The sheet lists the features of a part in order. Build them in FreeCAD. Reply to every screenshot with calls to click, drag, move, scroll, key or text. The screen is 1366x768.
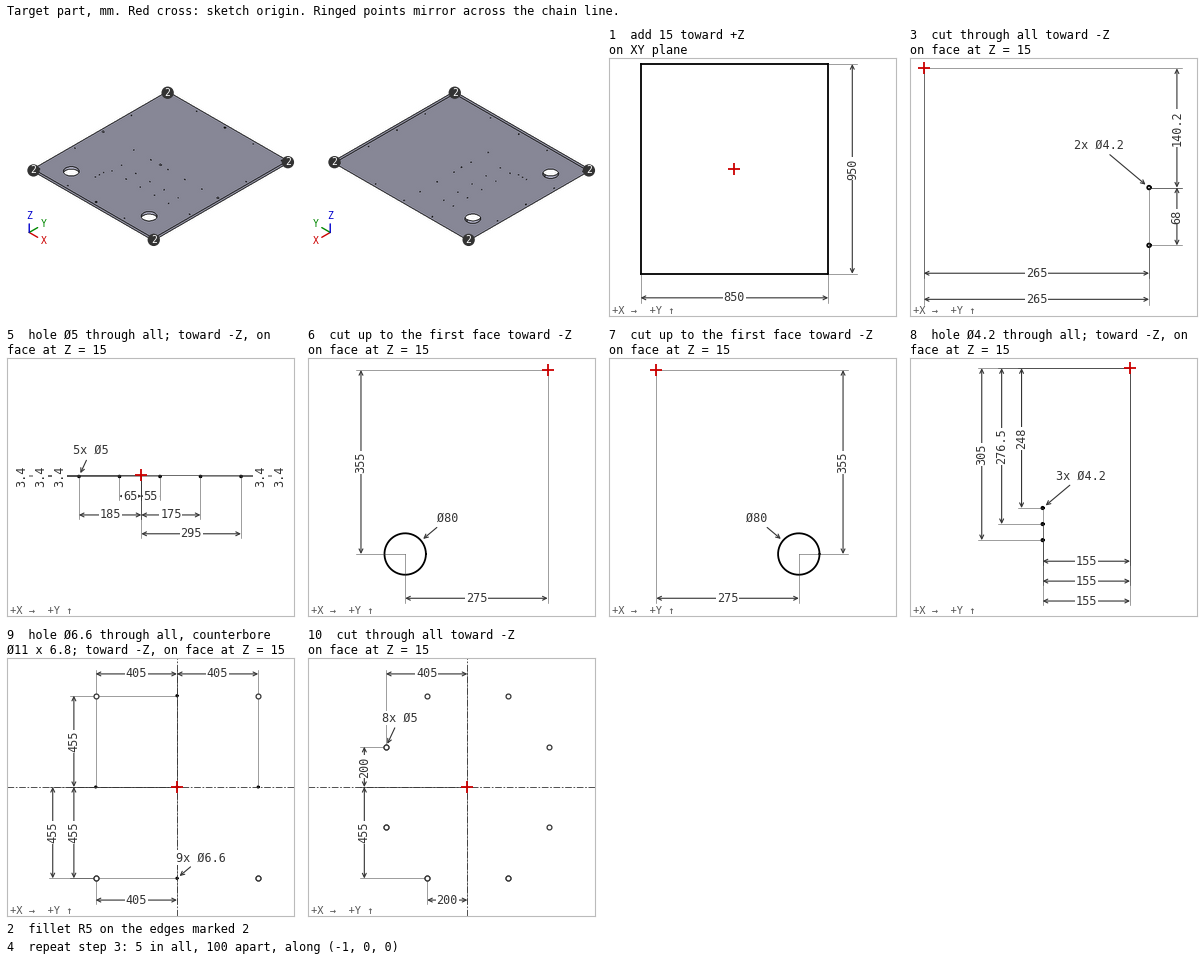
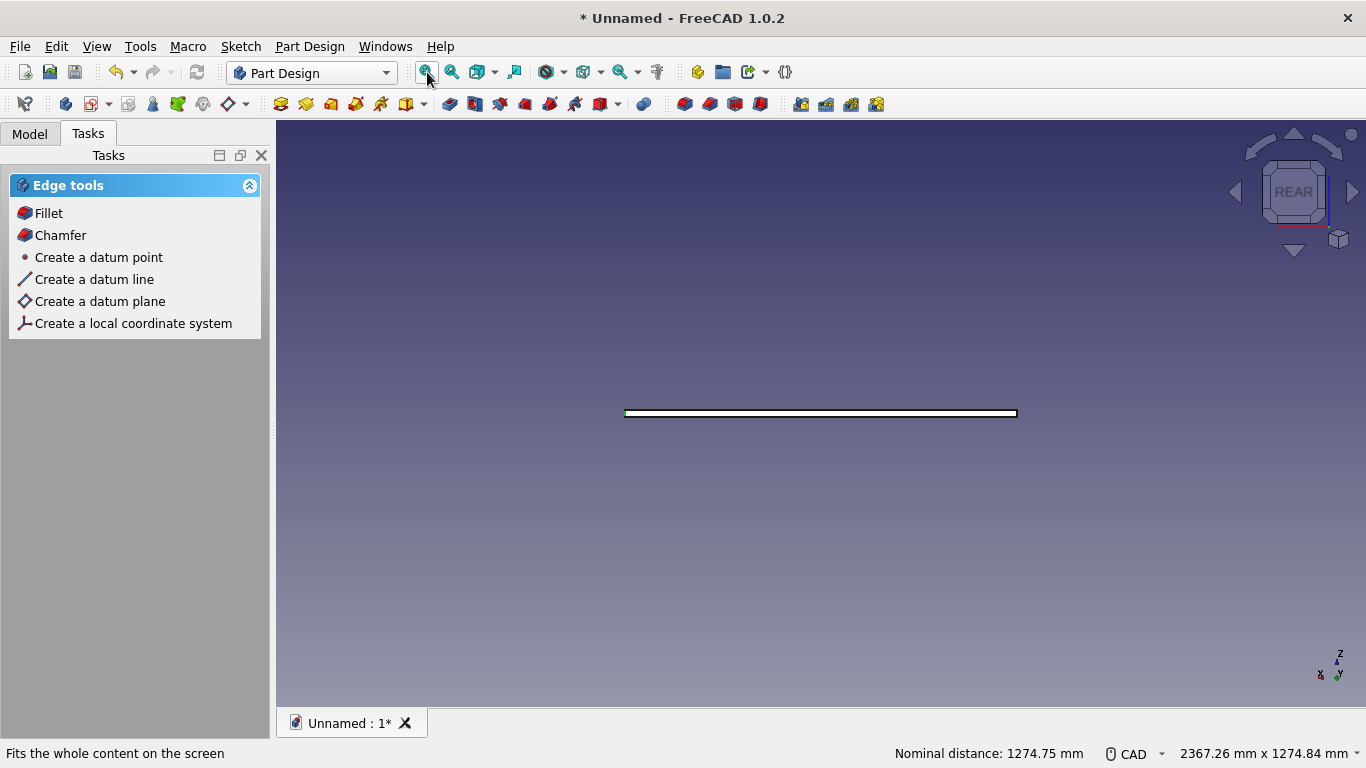
click(427, 72)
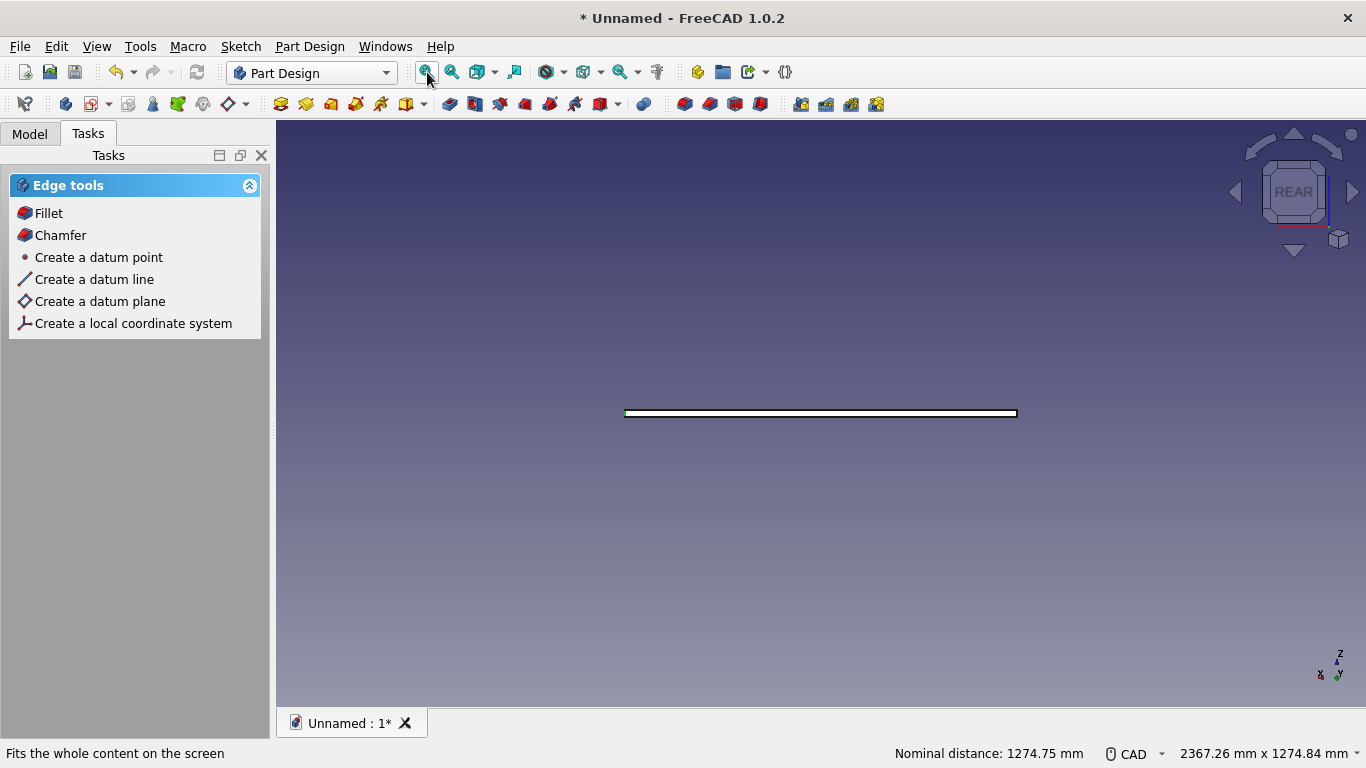
scroll(1017, 413, up, 9)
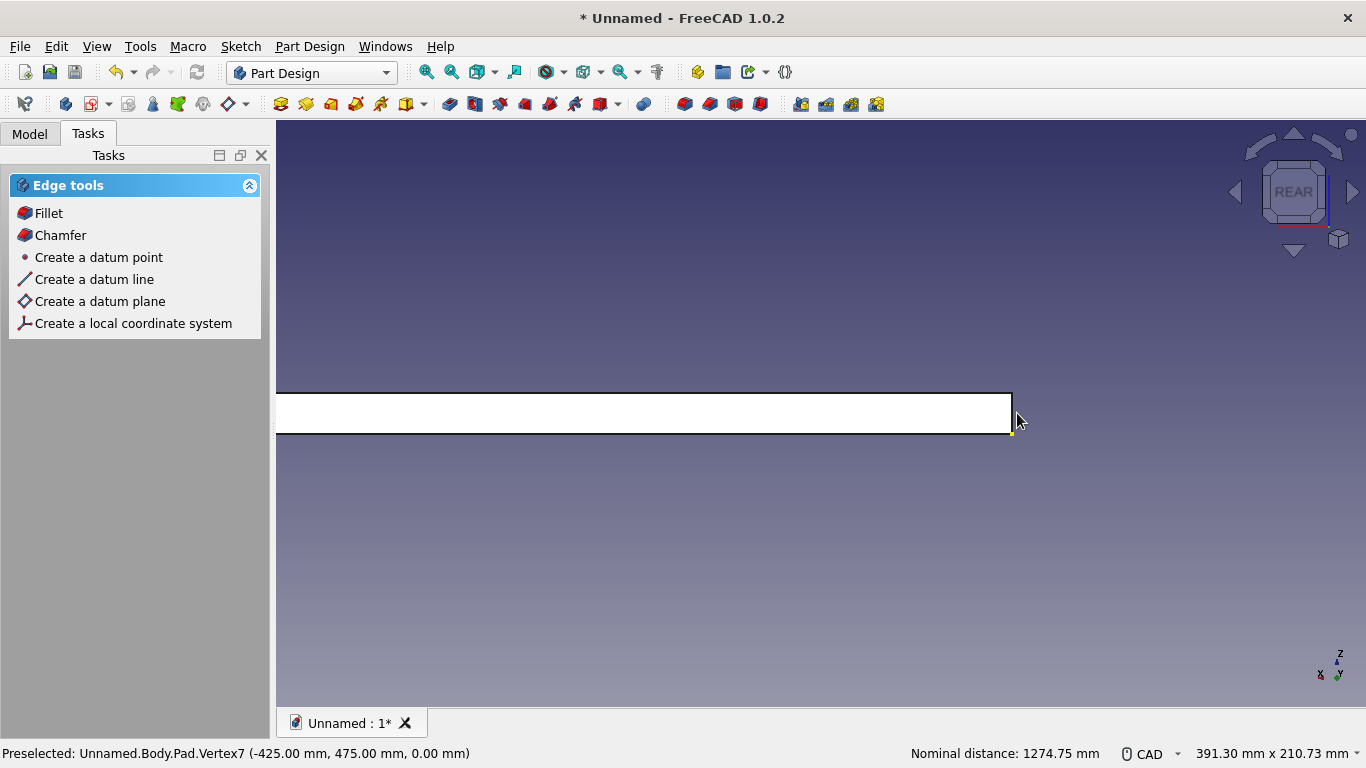
click(1012, 413, ctrl)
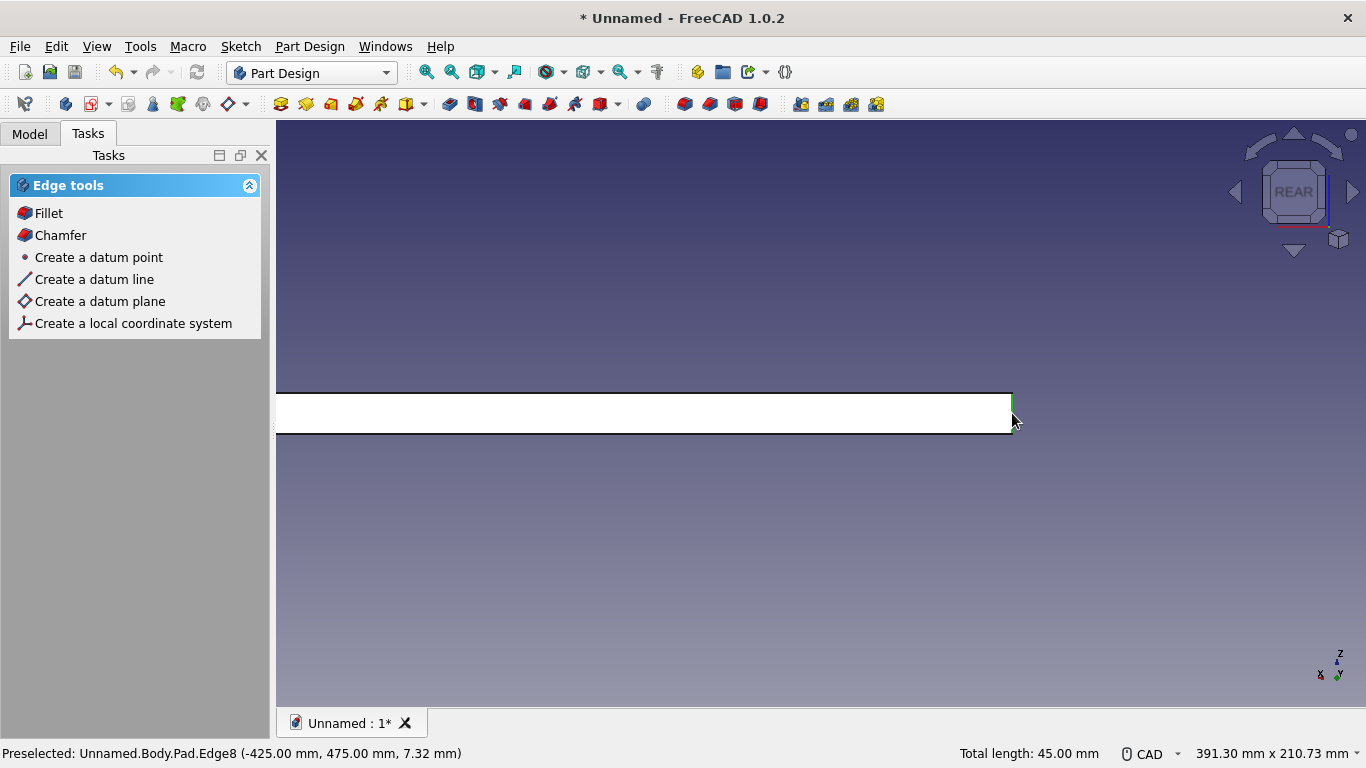
click(427, 72)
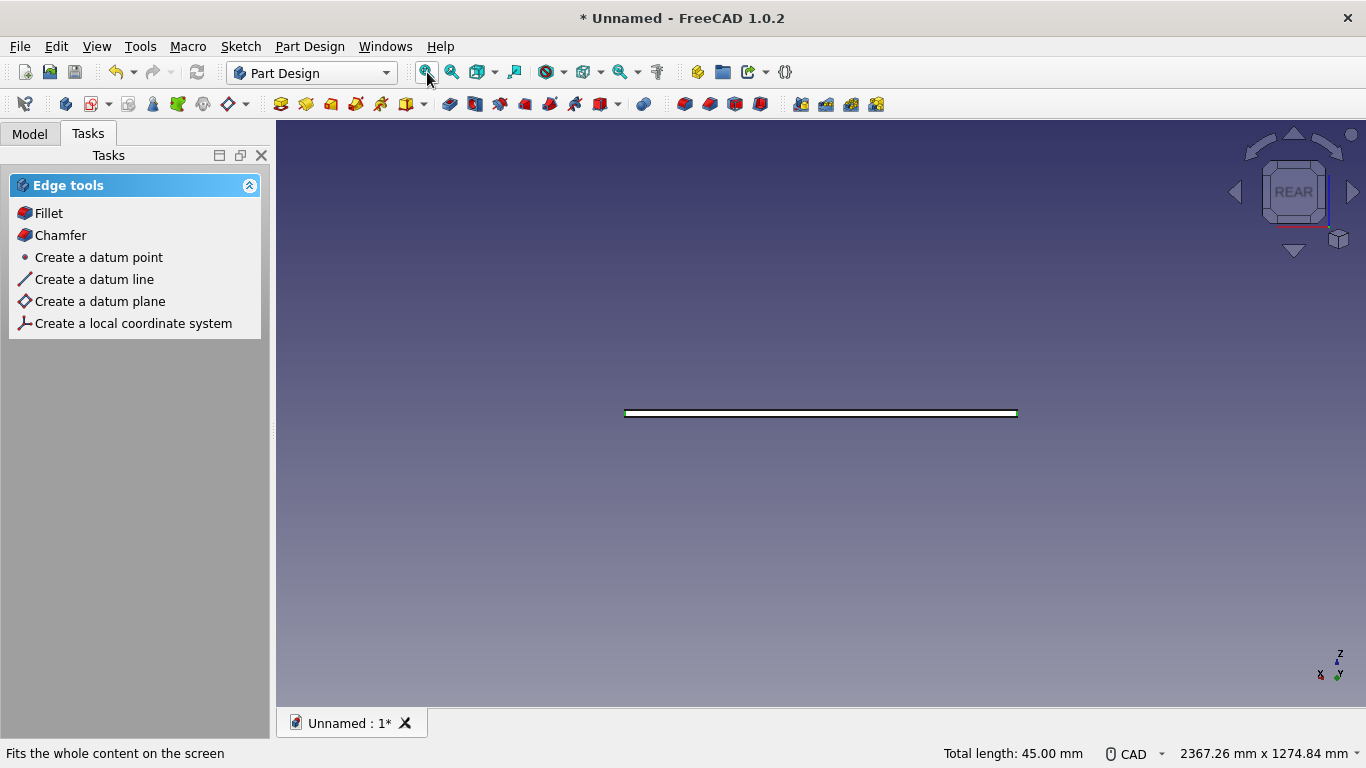
key(6)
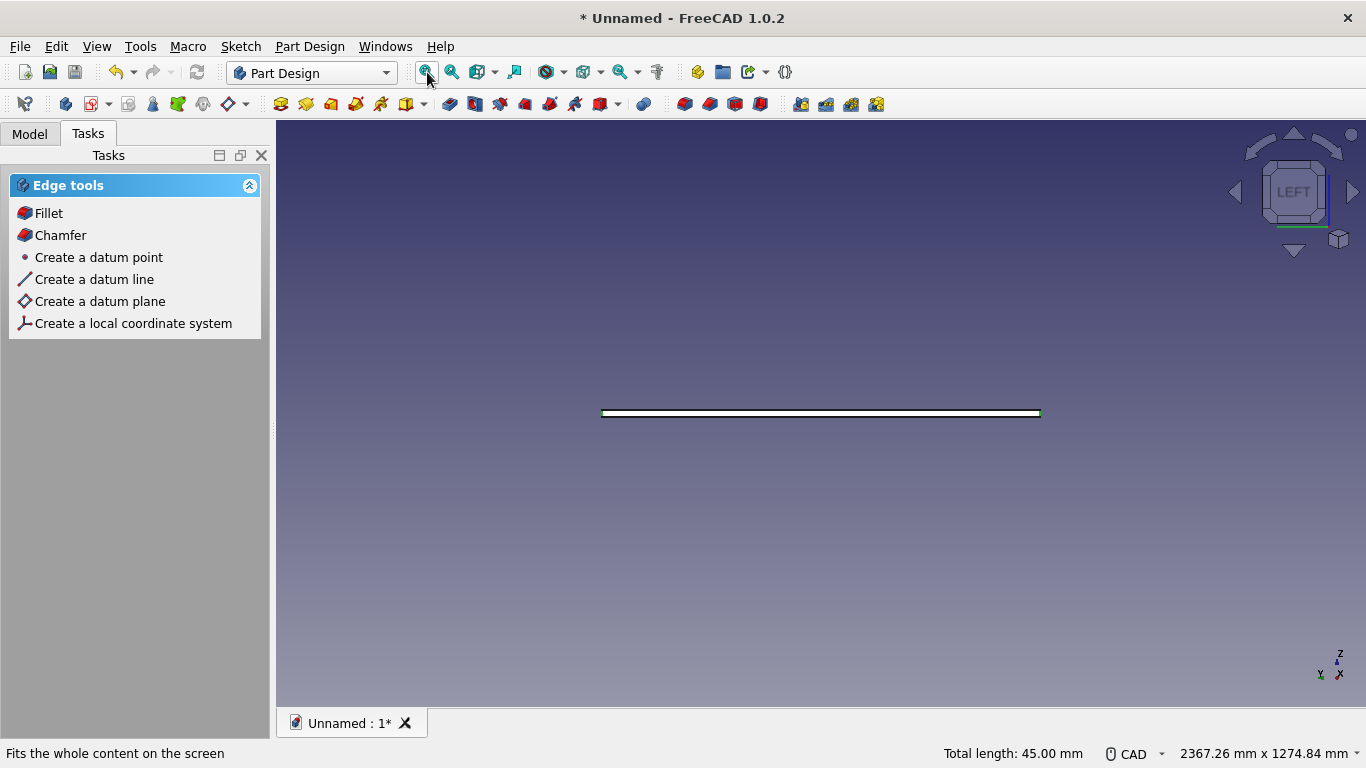
click(427, 72)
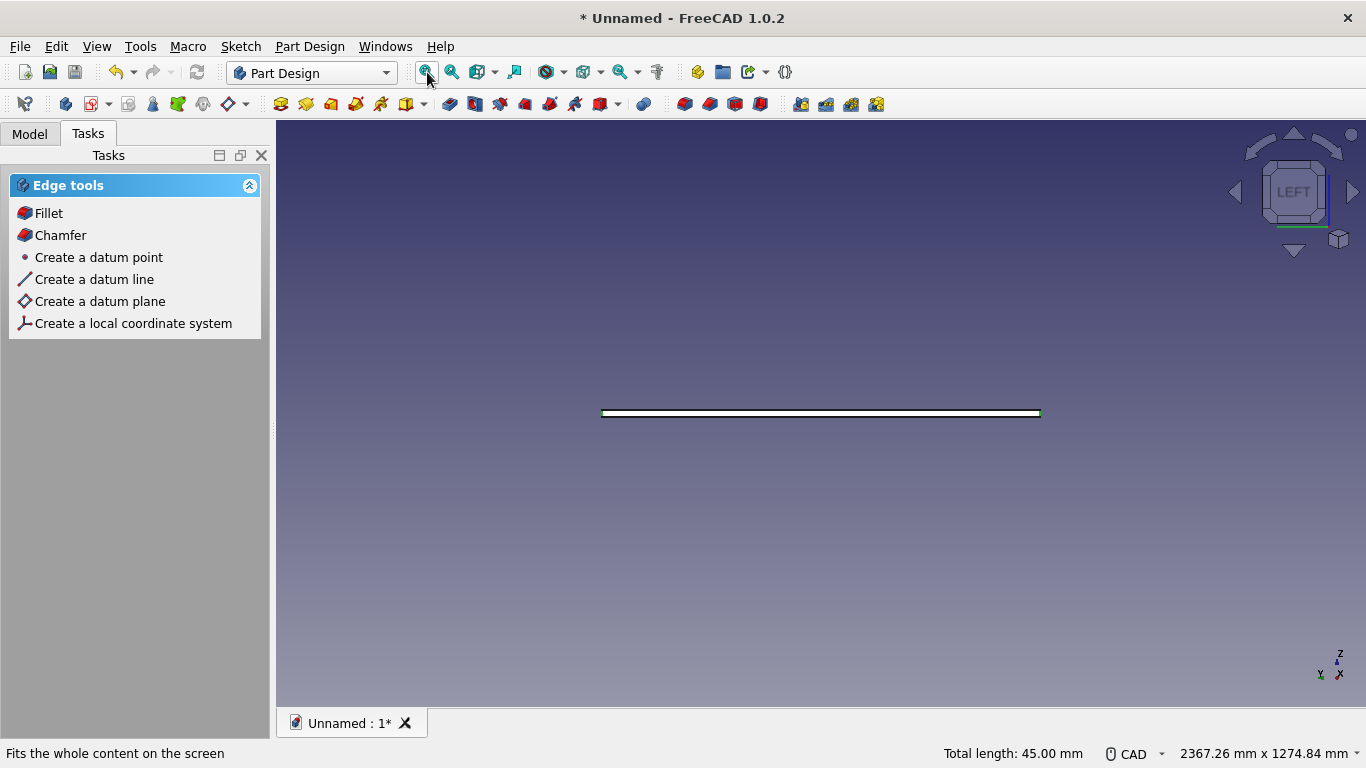
scroll(1040, 412, up, 9)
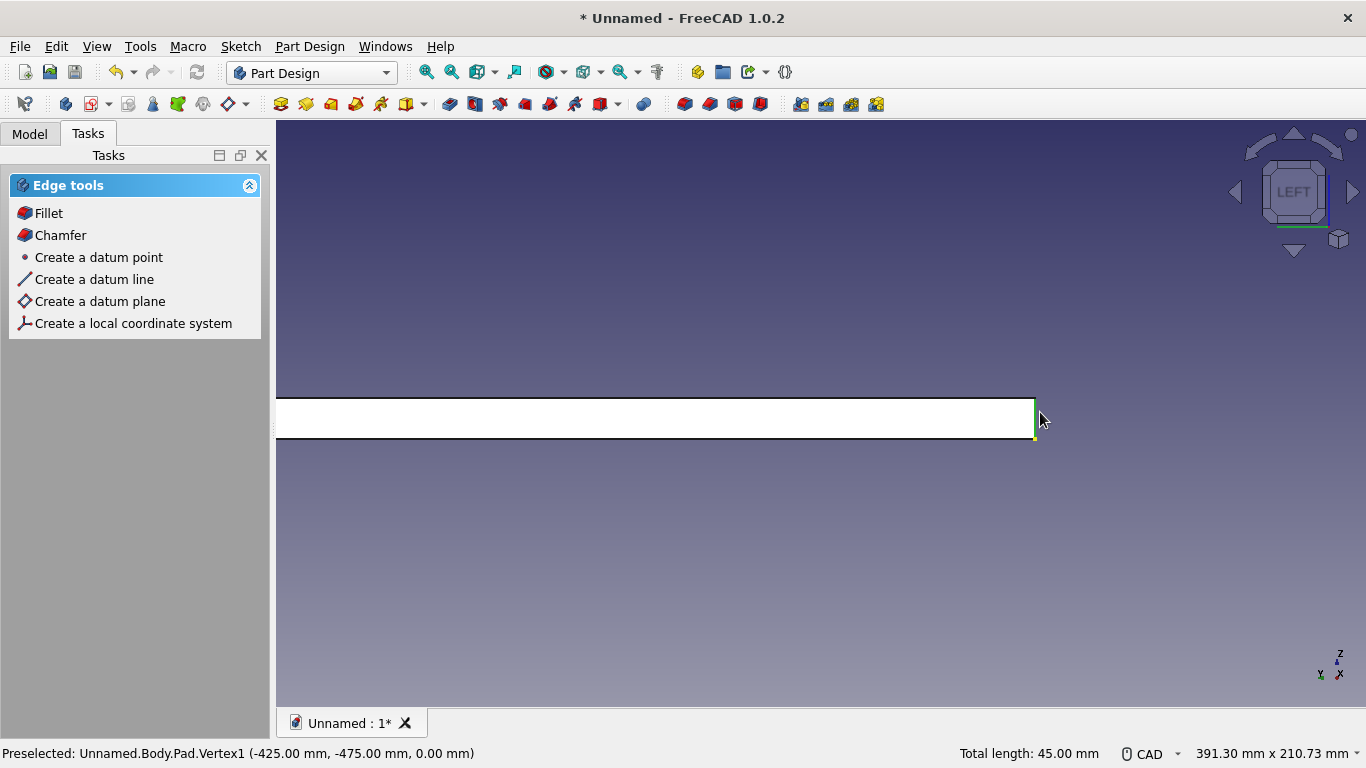
click(427, 72)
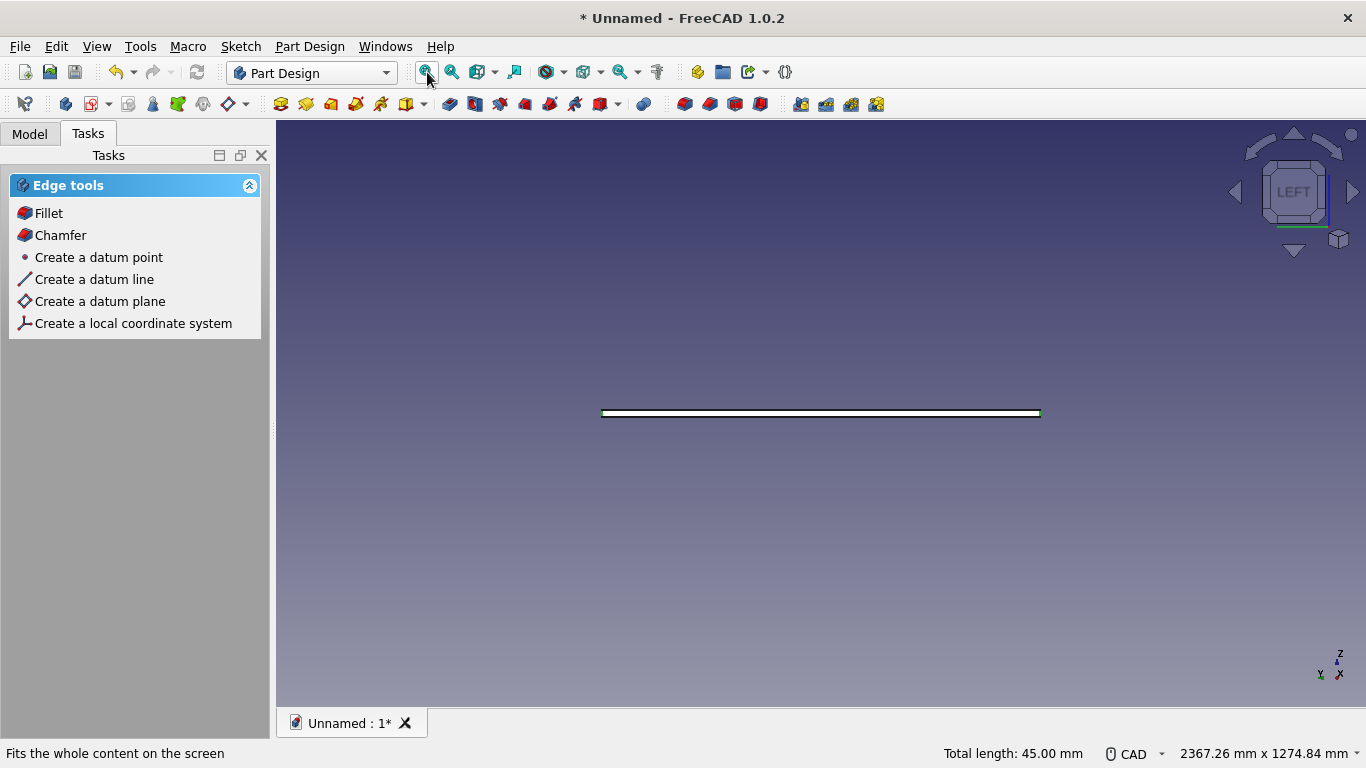
key(v)
key(3)